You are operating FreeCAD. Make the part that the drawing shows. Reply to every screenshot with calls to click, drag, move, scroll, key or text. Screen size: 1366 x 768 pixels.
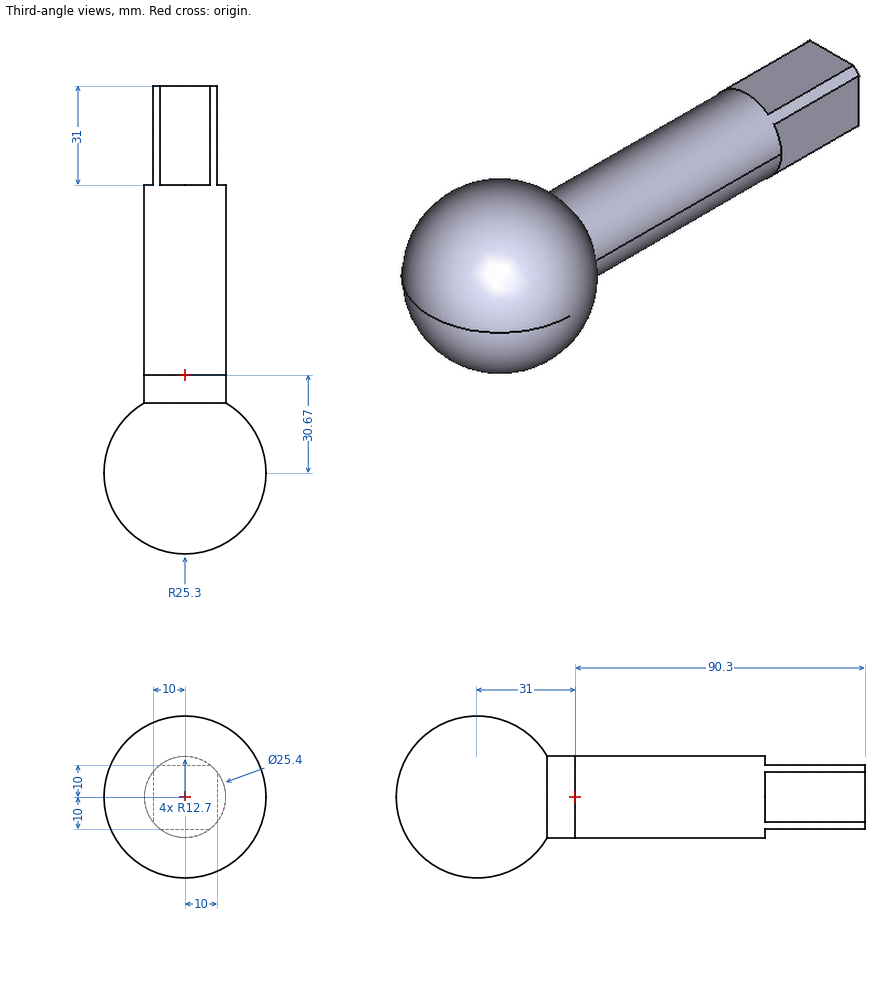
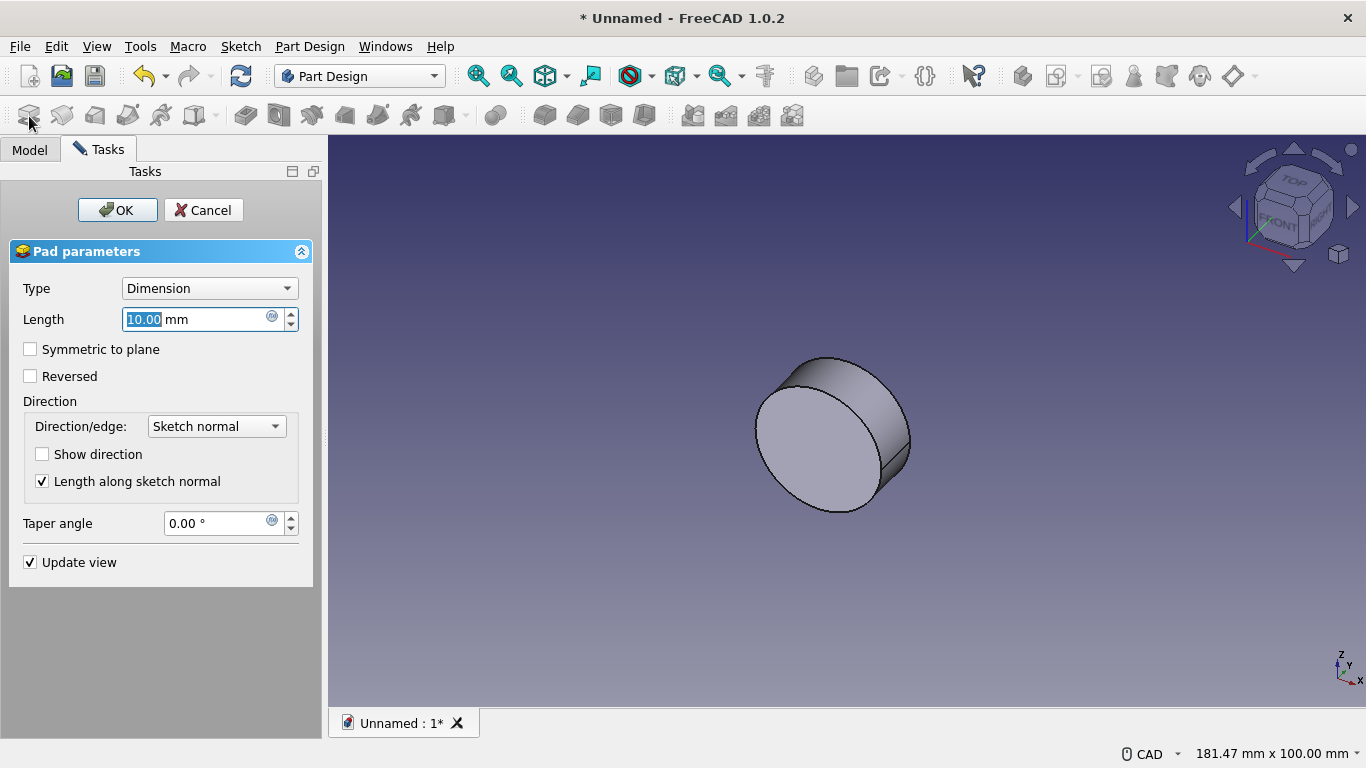
text(90.3)
key(Tab)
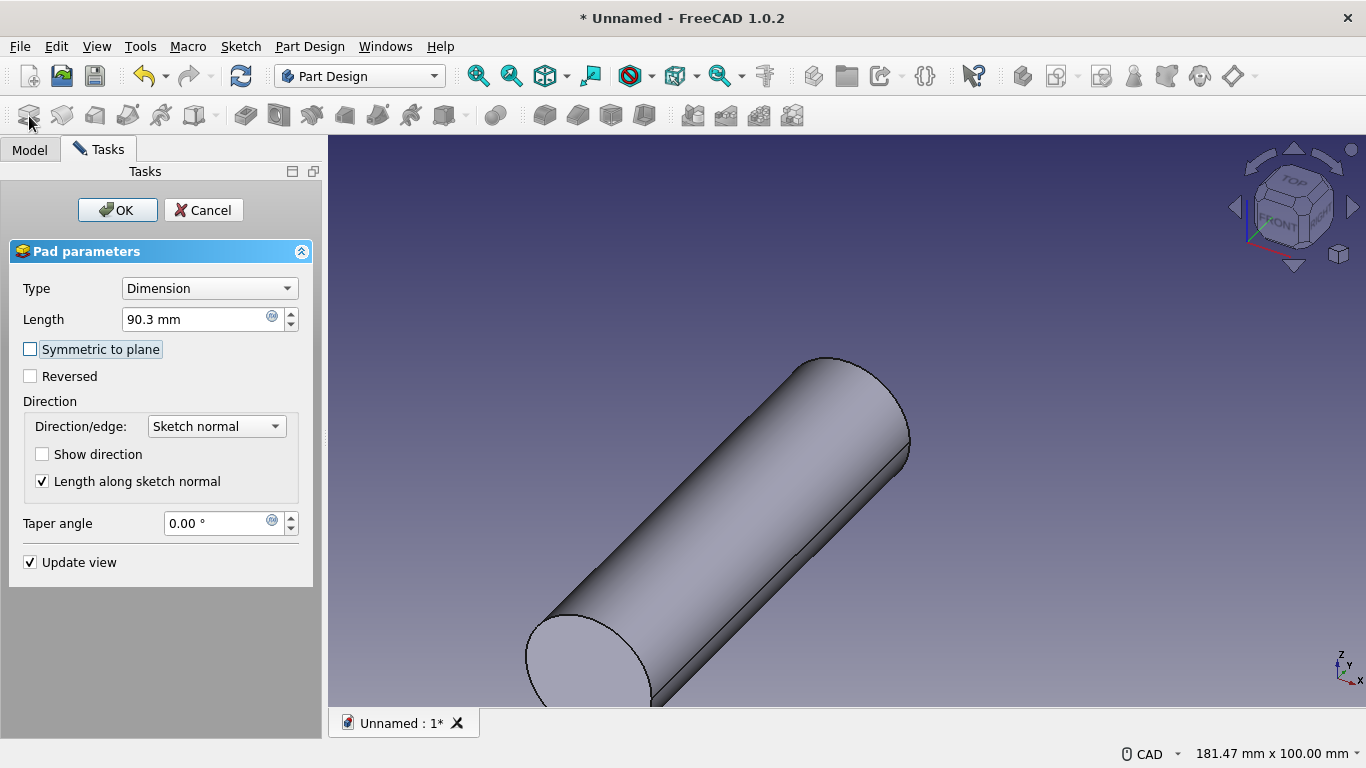
click(31, 376)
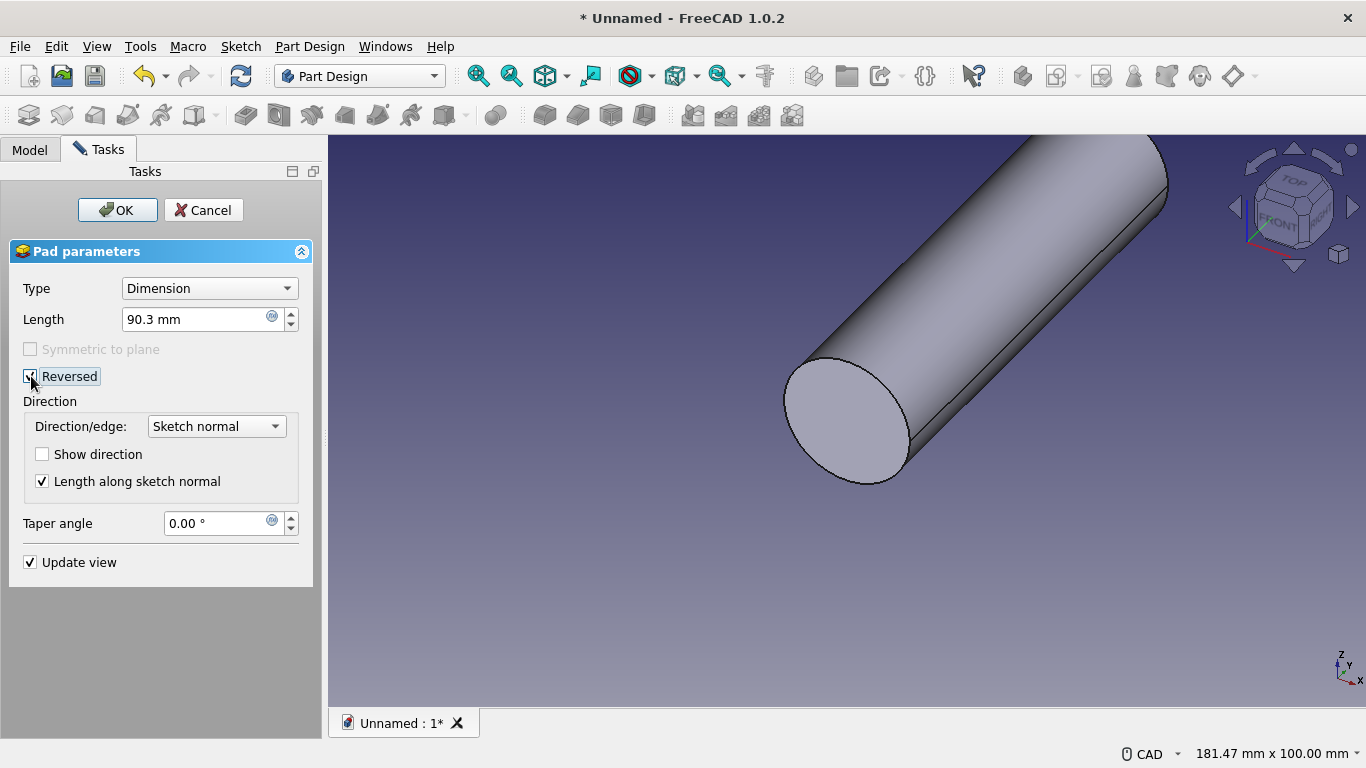
click(118, 210)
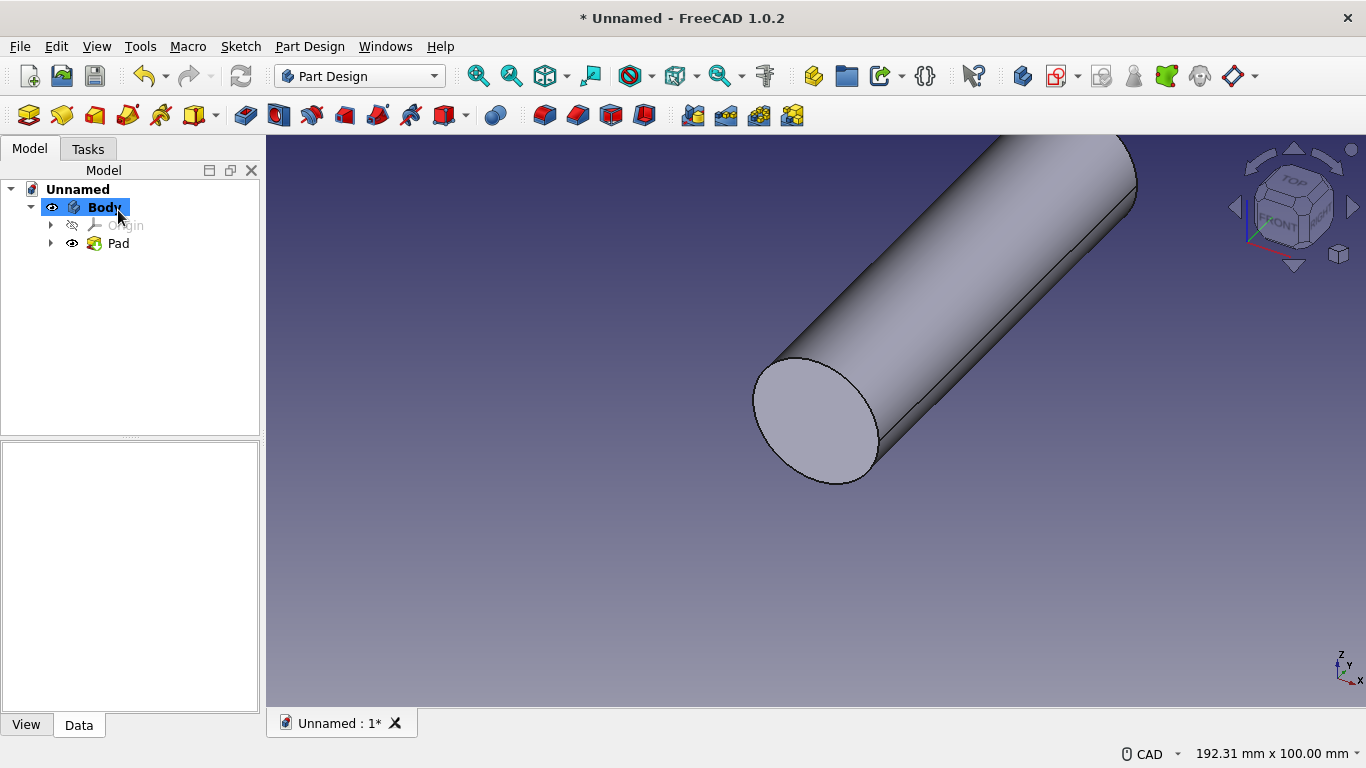
click(479, 76)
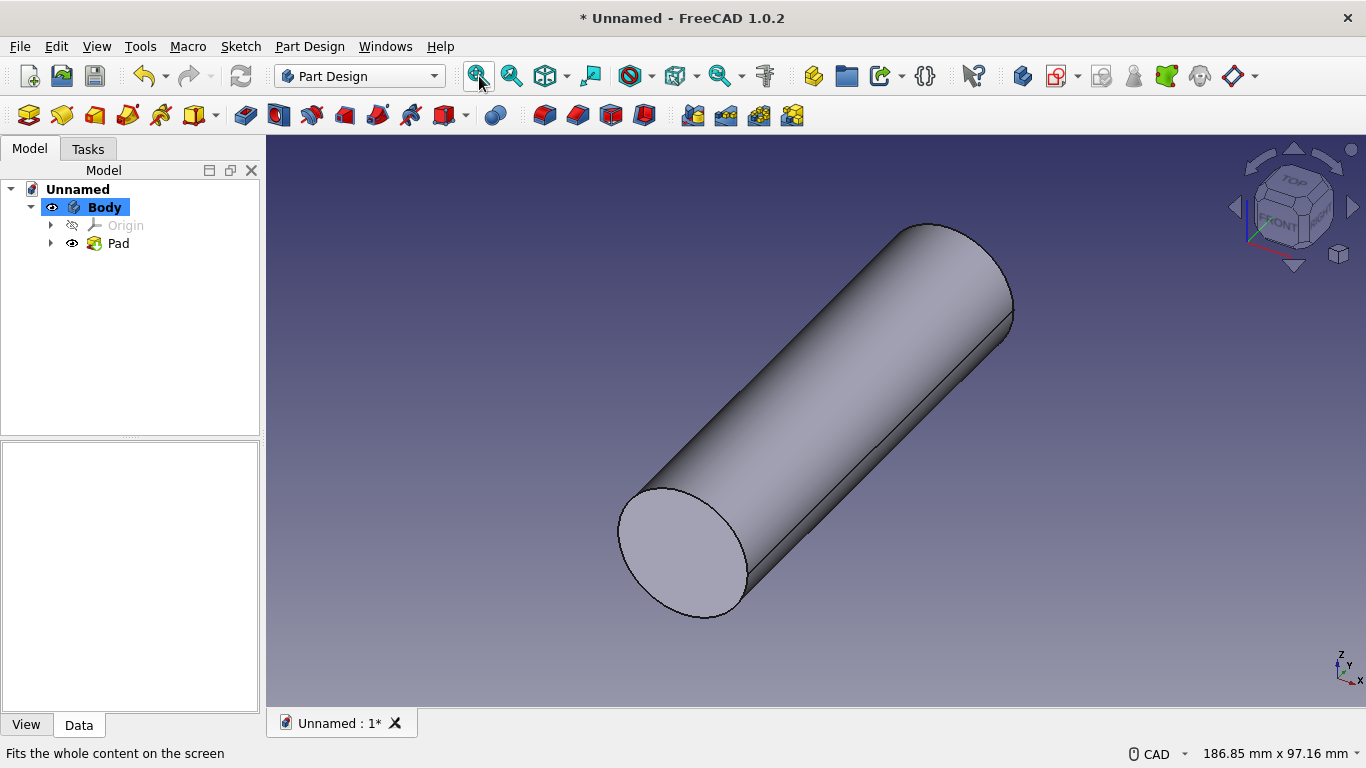
click(51, 225)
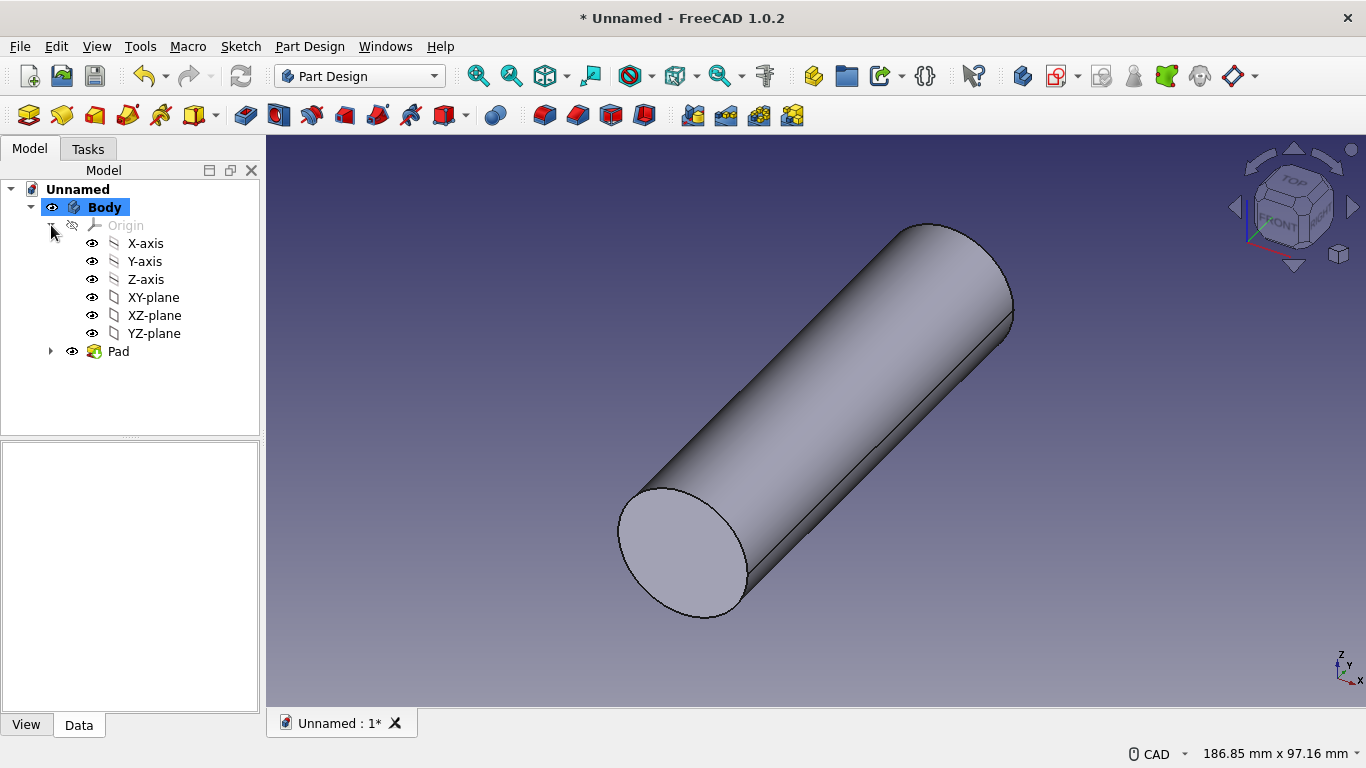
click(137, 315)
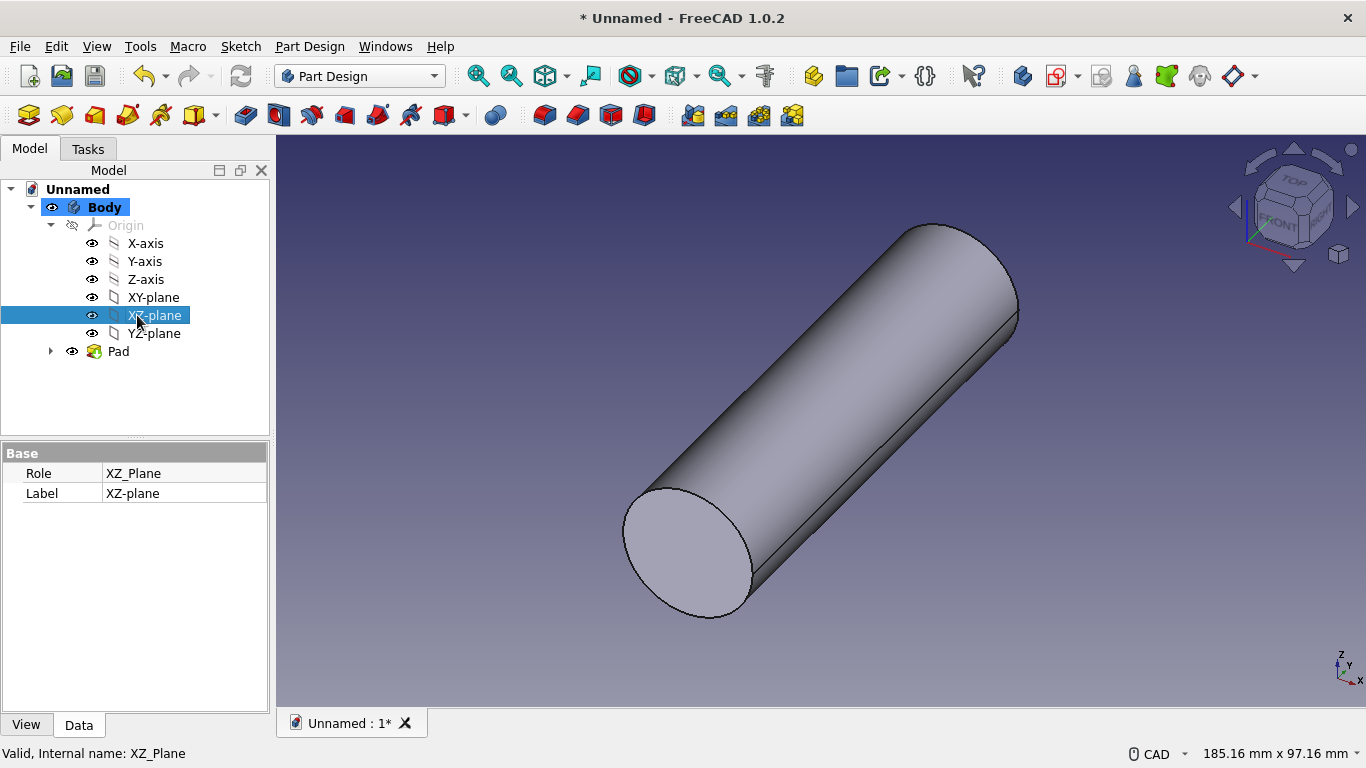
click(1232, 76)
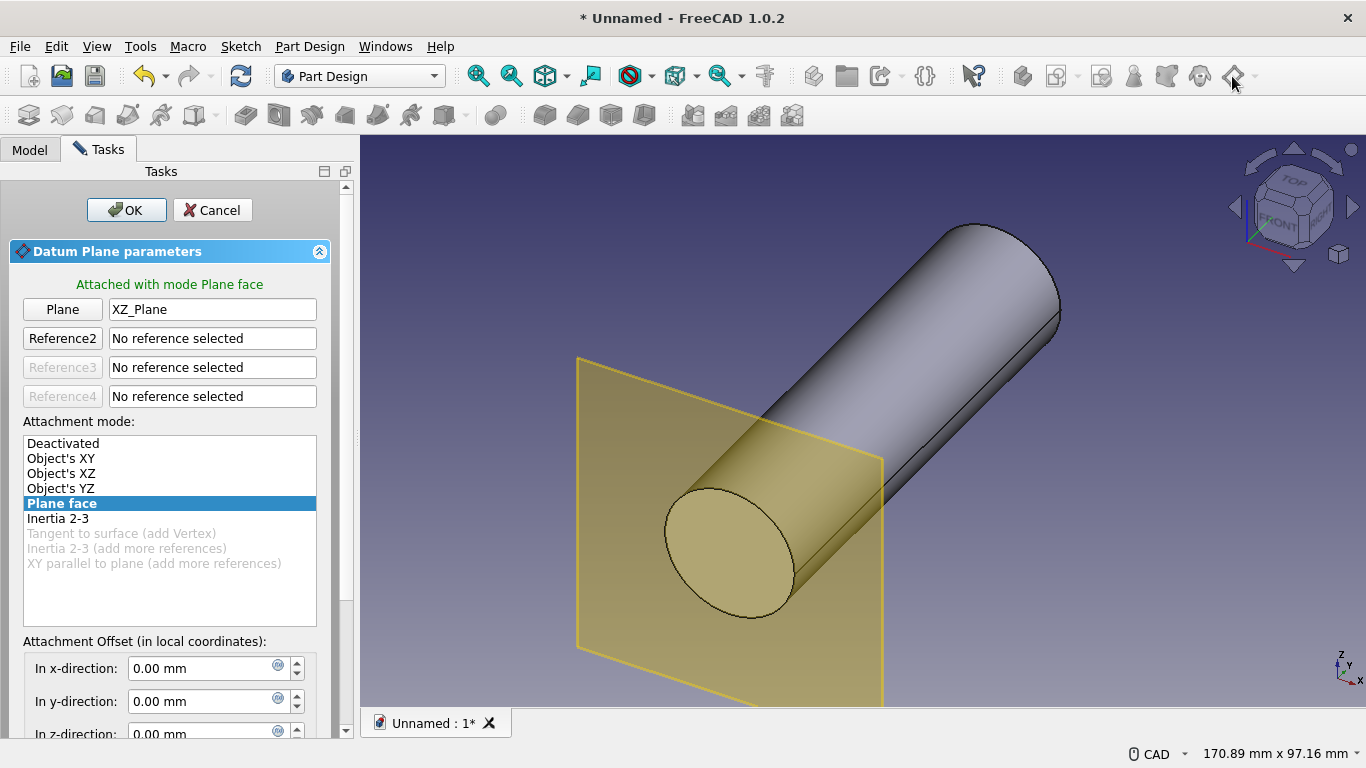
scroll(346, 460, down, 2)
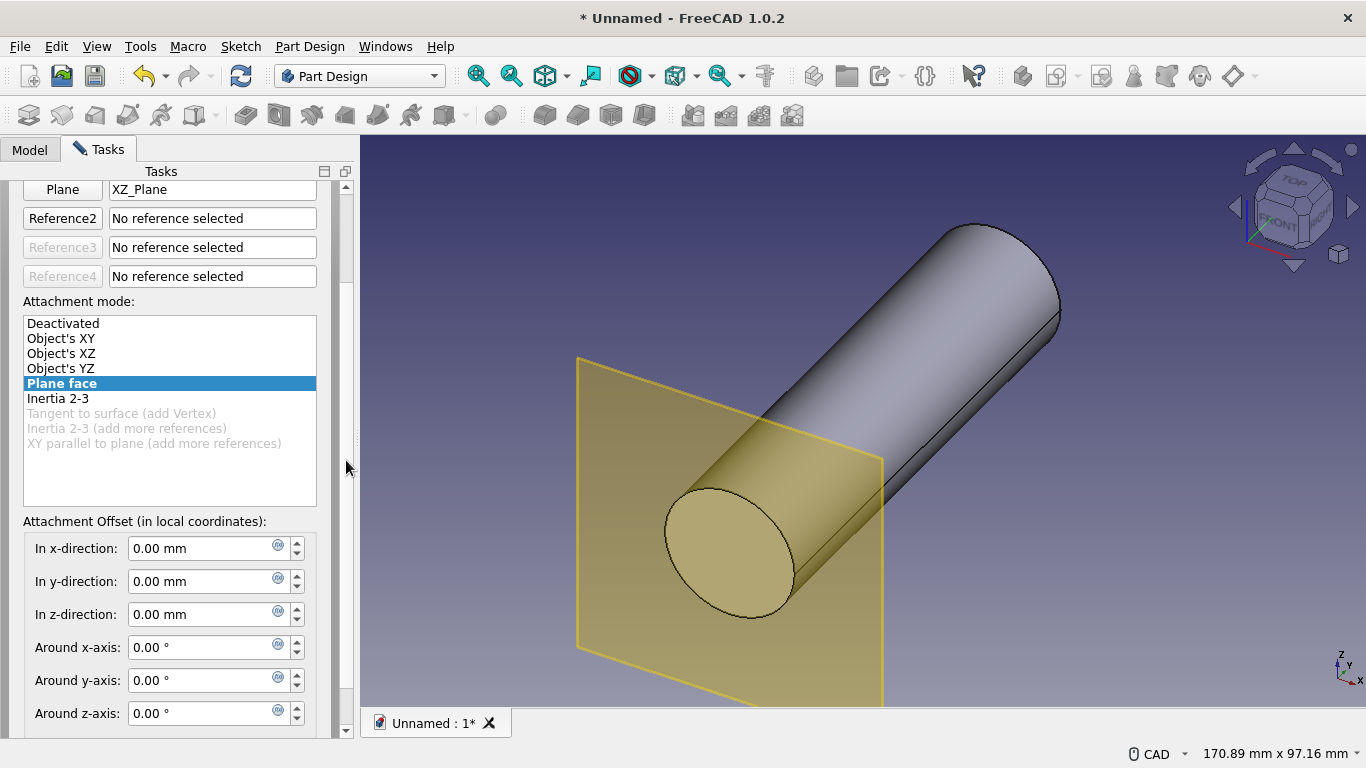
triple_click(210, 614)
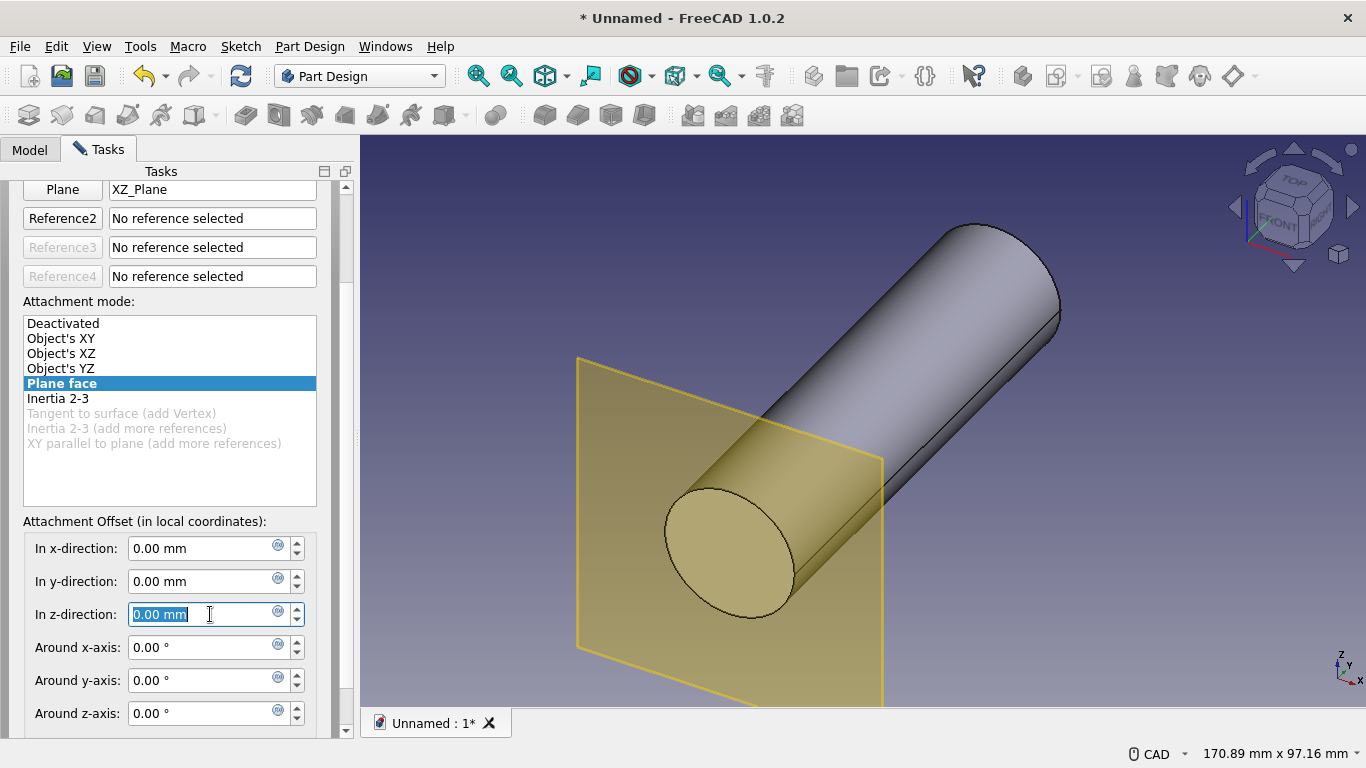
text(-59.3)
key(Tab)